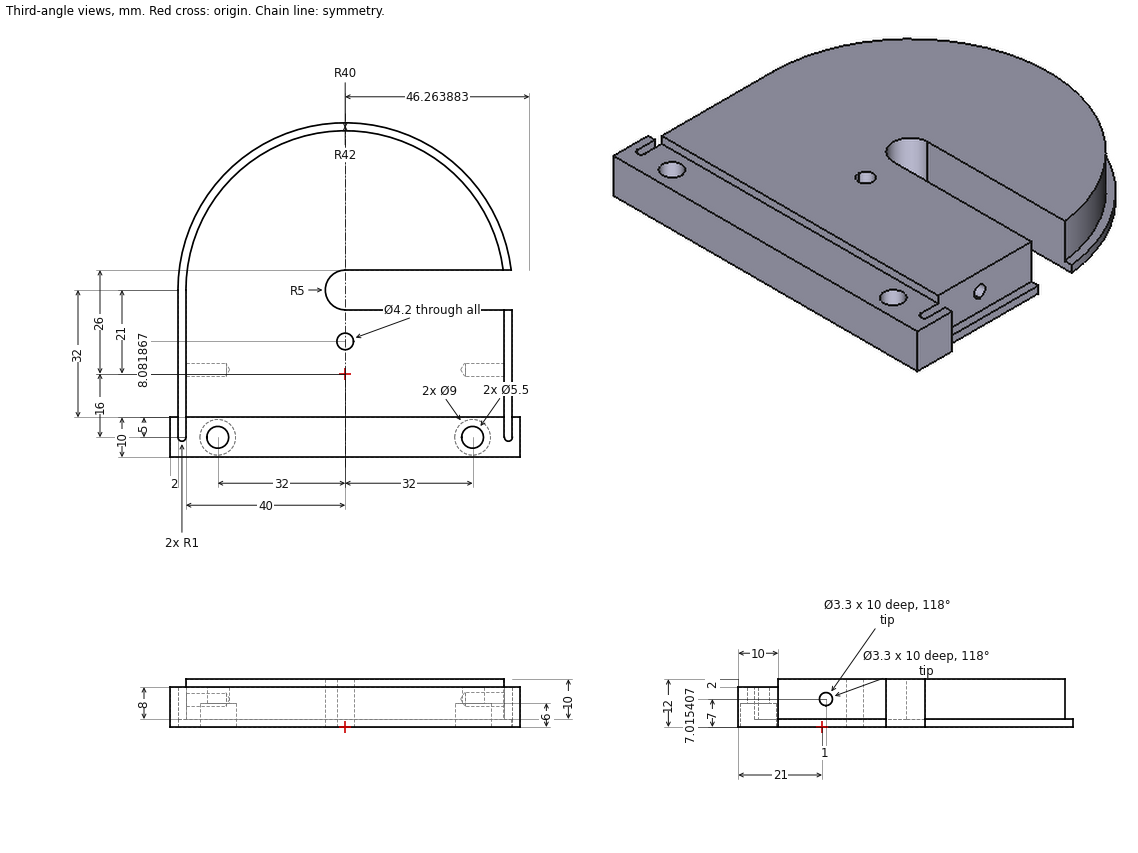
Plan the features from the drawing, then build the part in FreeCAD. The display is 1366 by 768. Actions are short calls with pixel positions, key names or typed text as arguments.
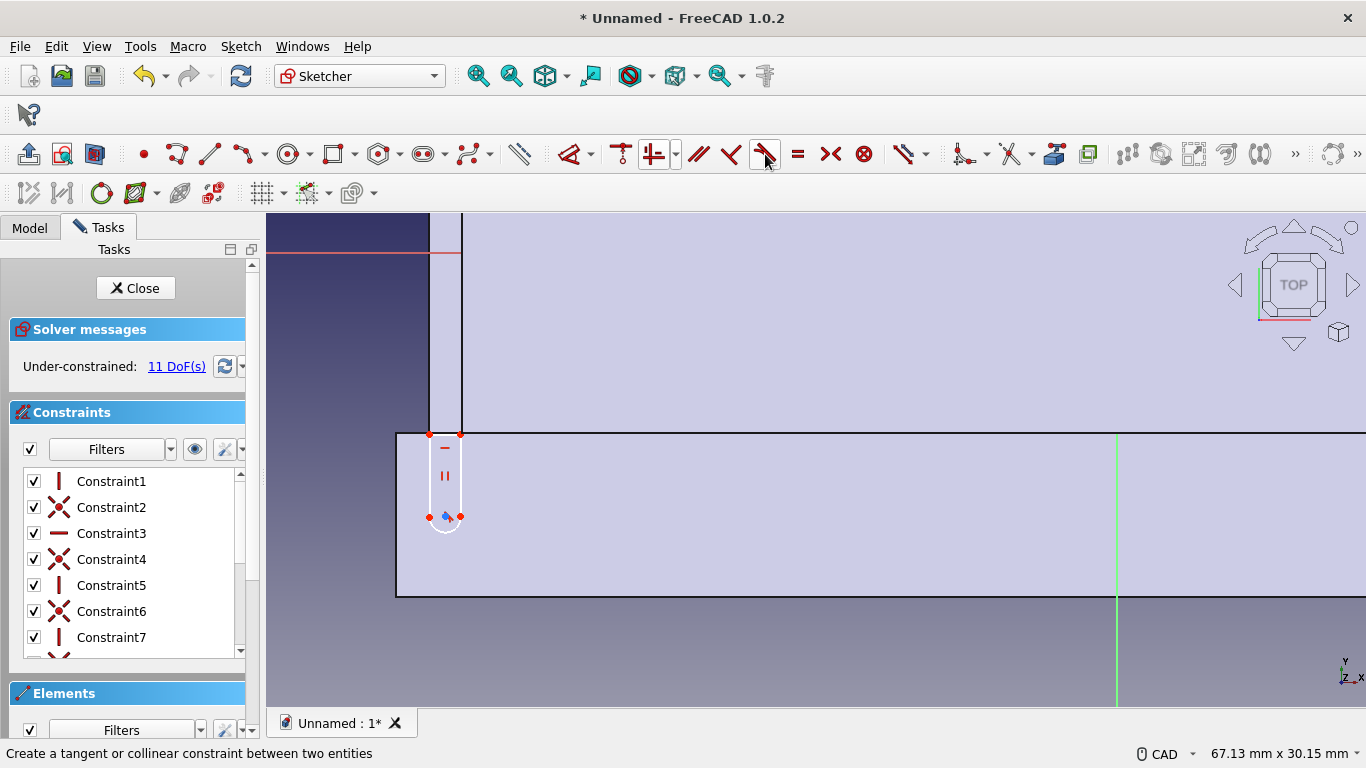
click(430, 460)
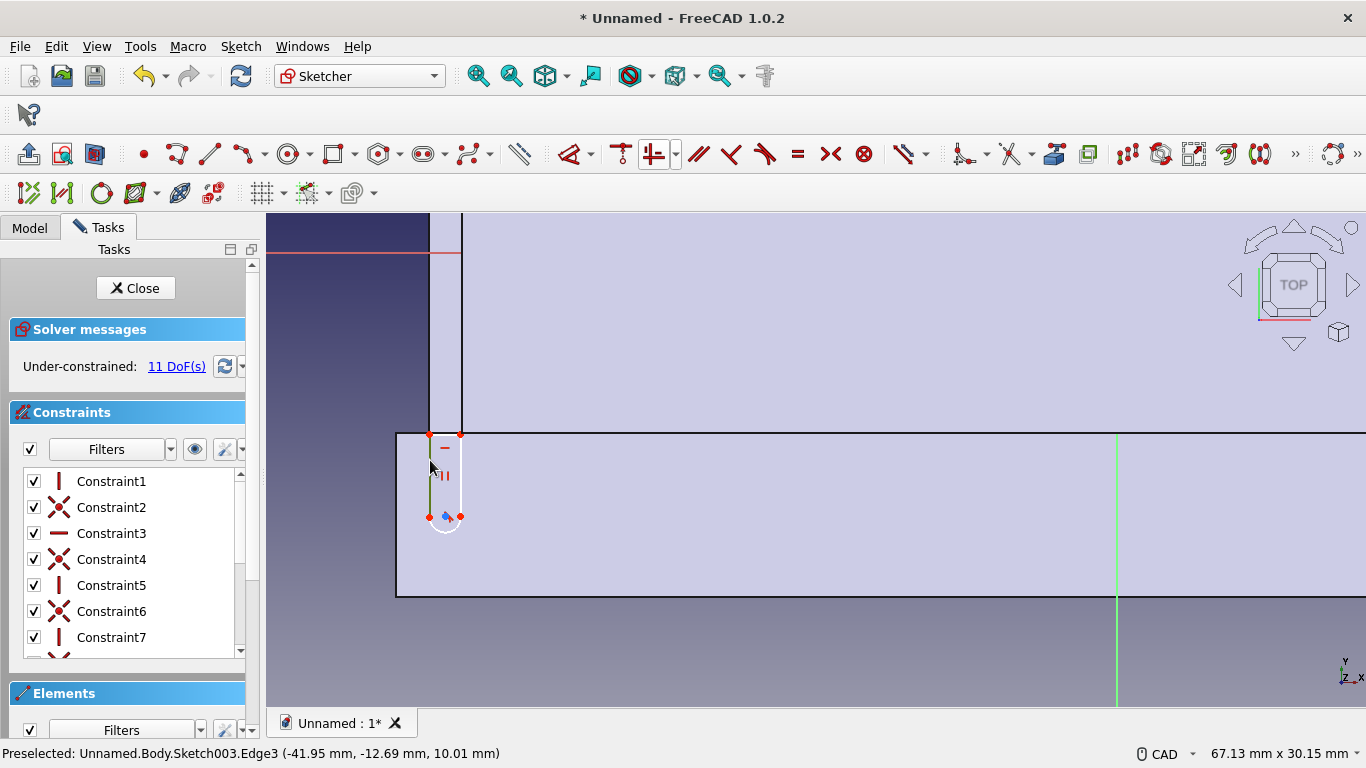
click(436, 530)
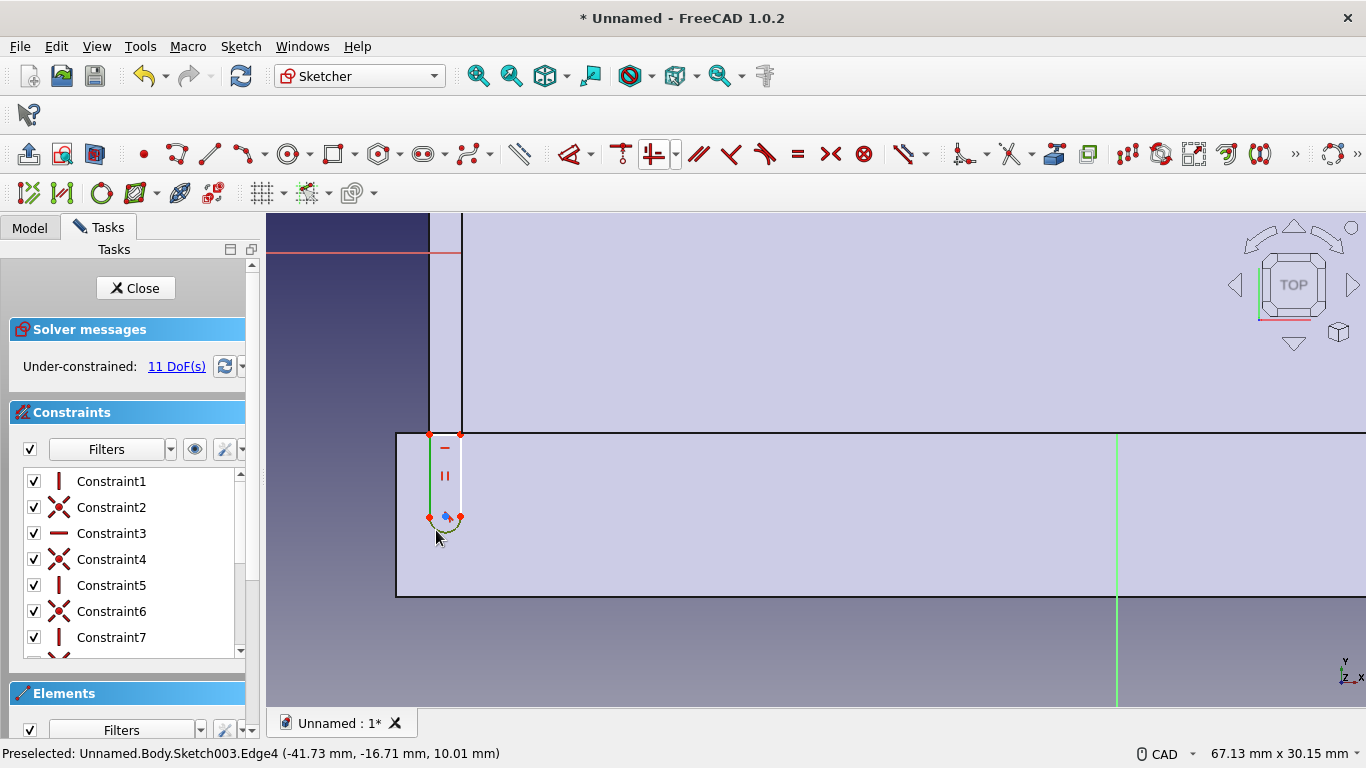
click(765, 154)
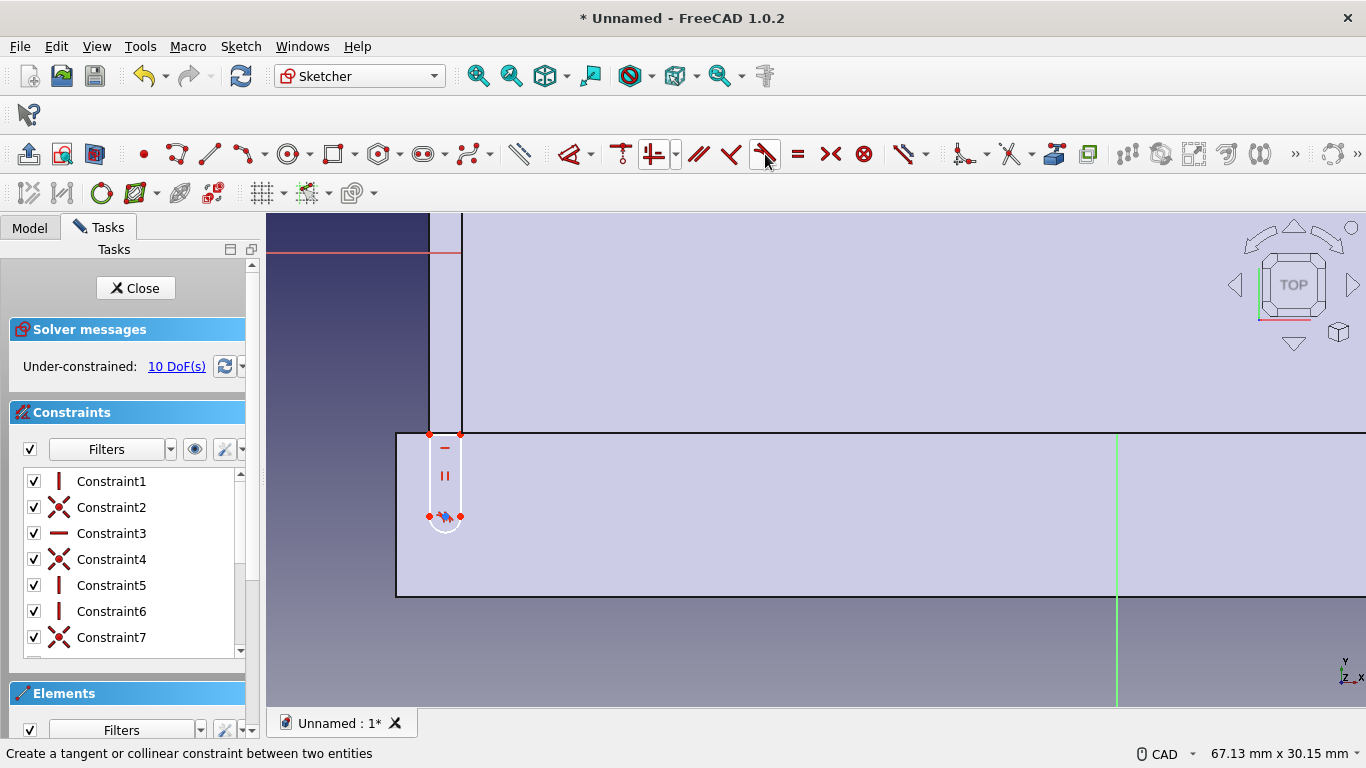
scroll(446, 515, down, 4)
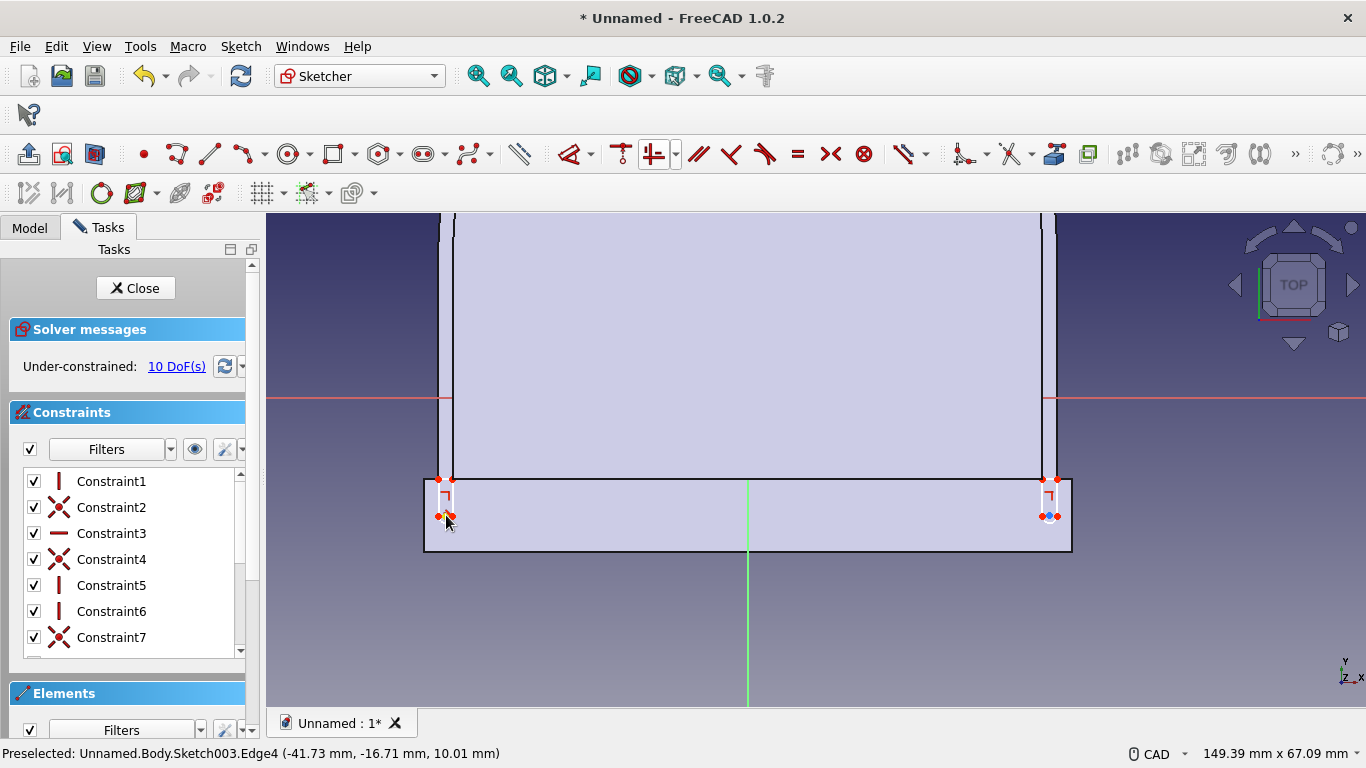
scroll(1057, 505, up, 2)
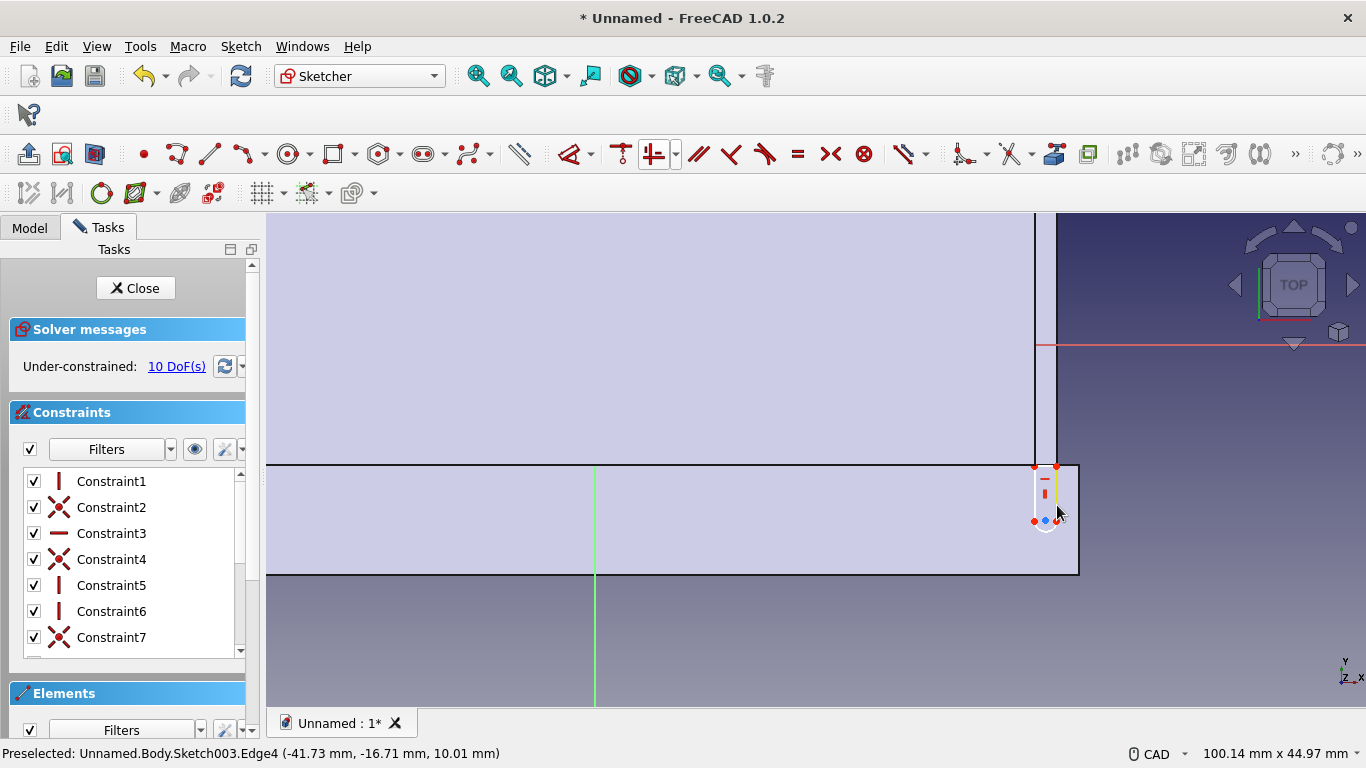
click(1057, 505)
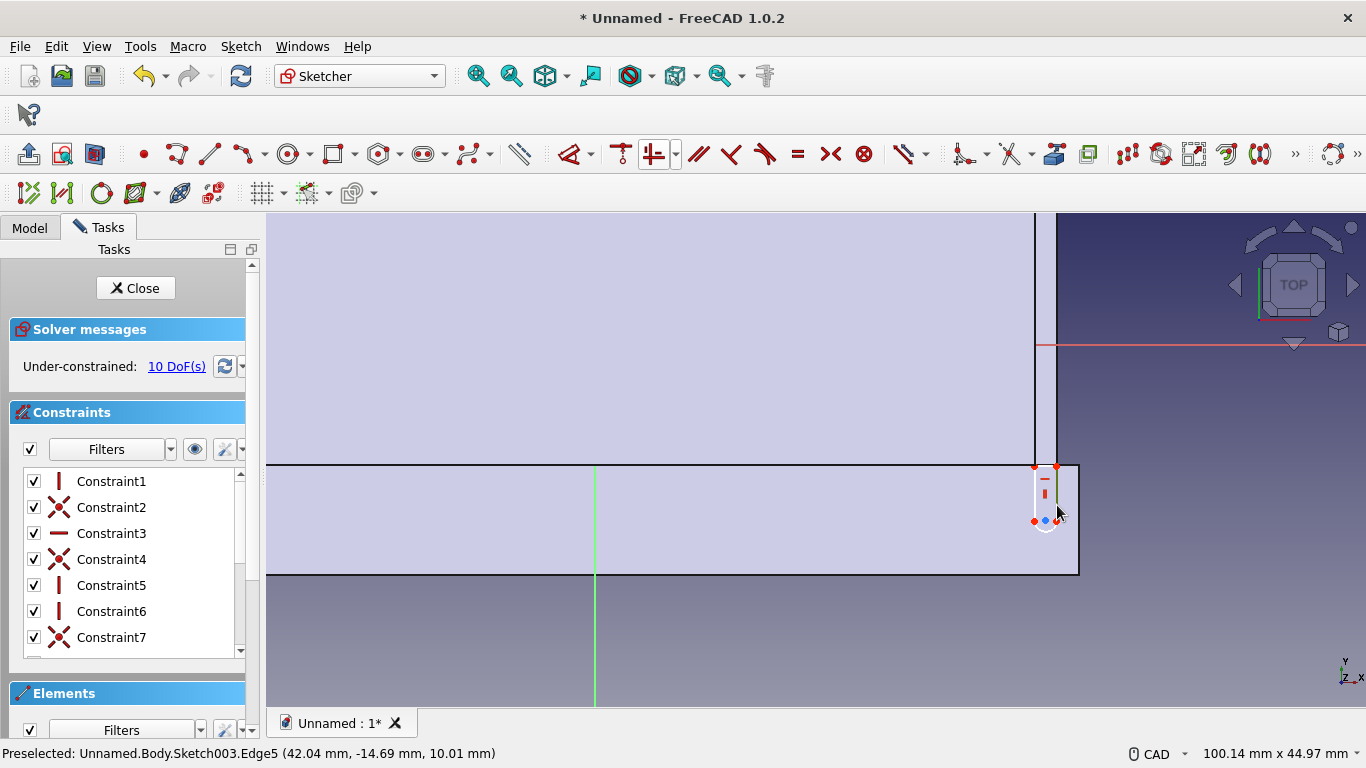
scroll(1040, 530, up, 2)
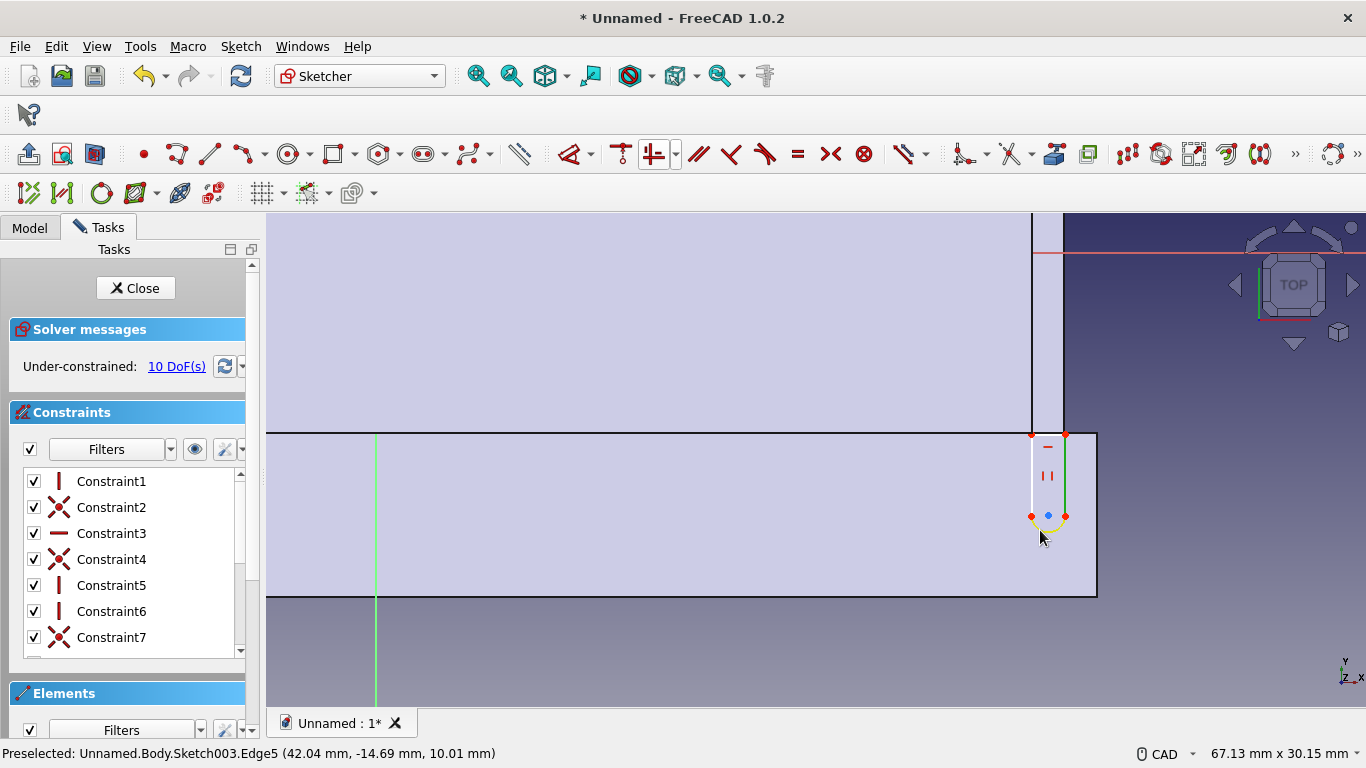
click(1039, 529)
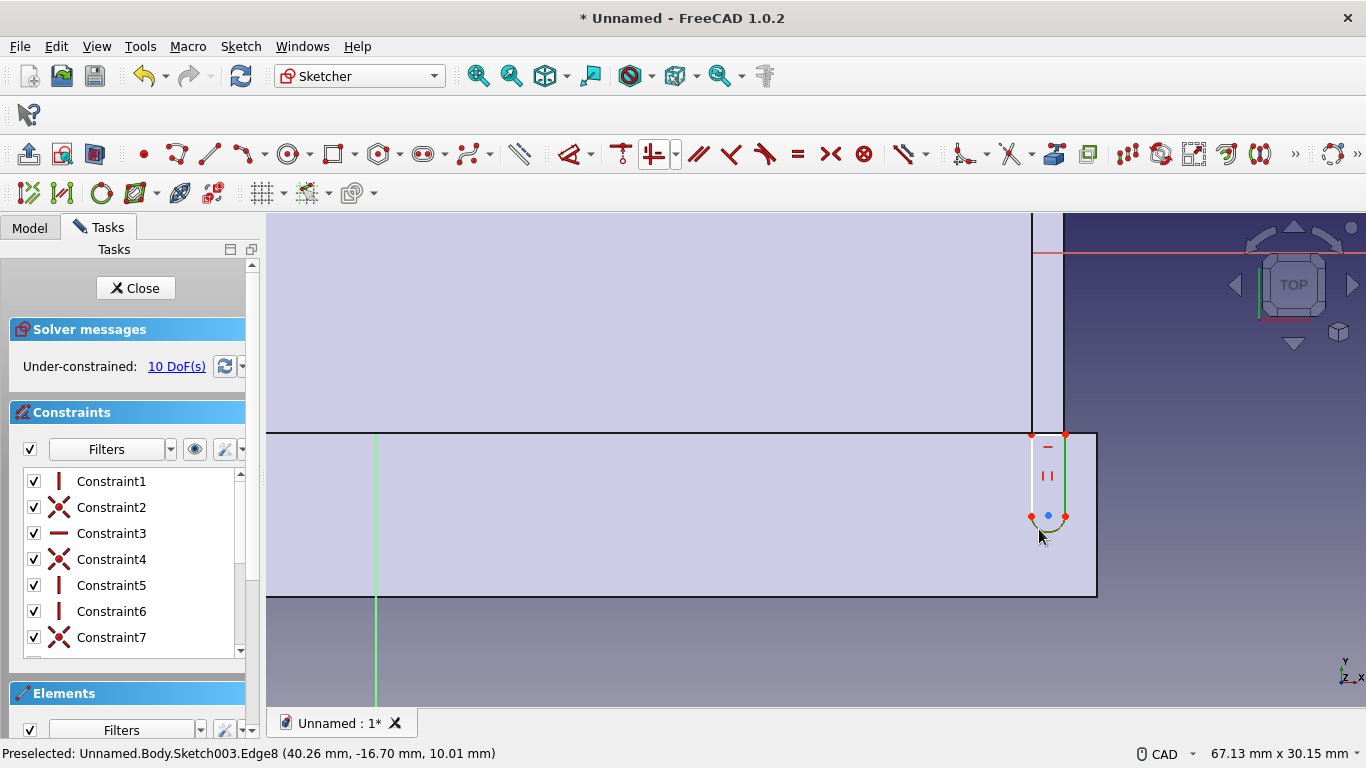
click(765, 154)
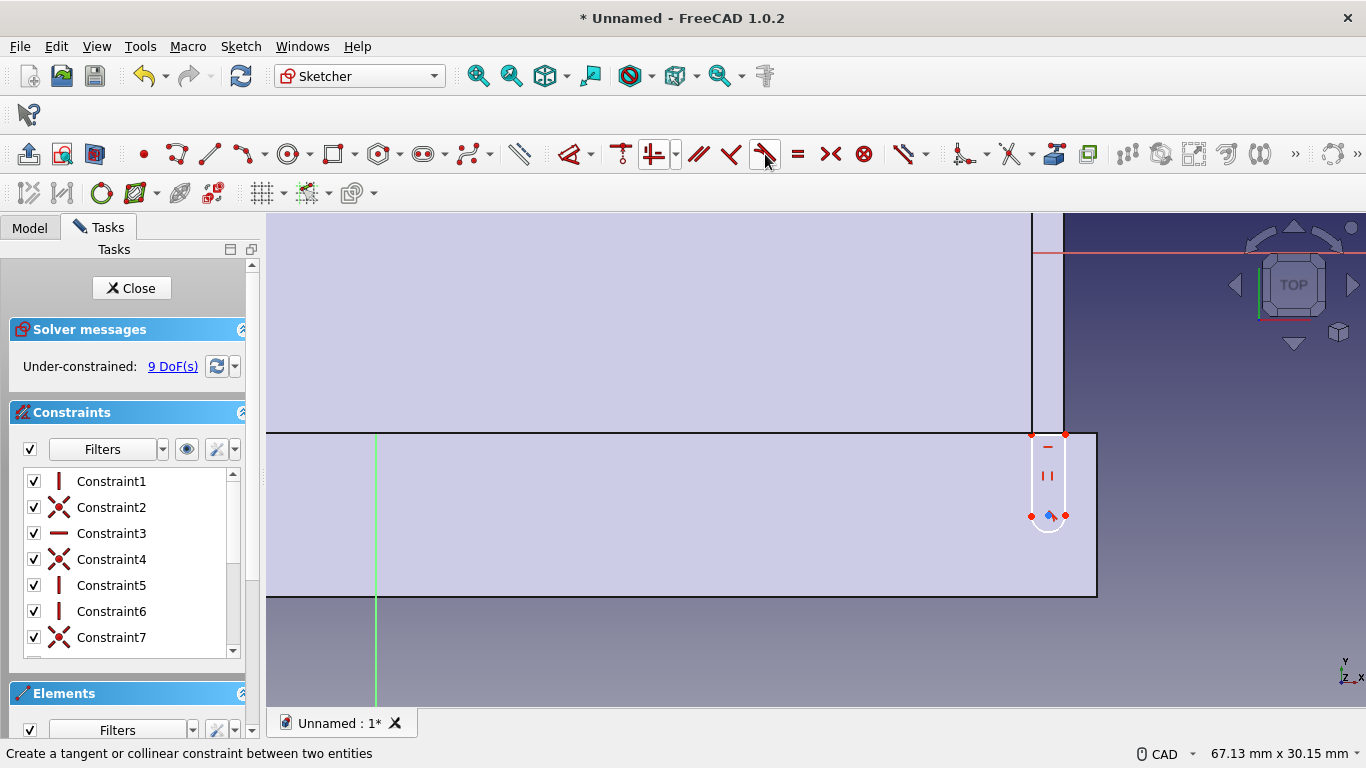
click(1032, 459)